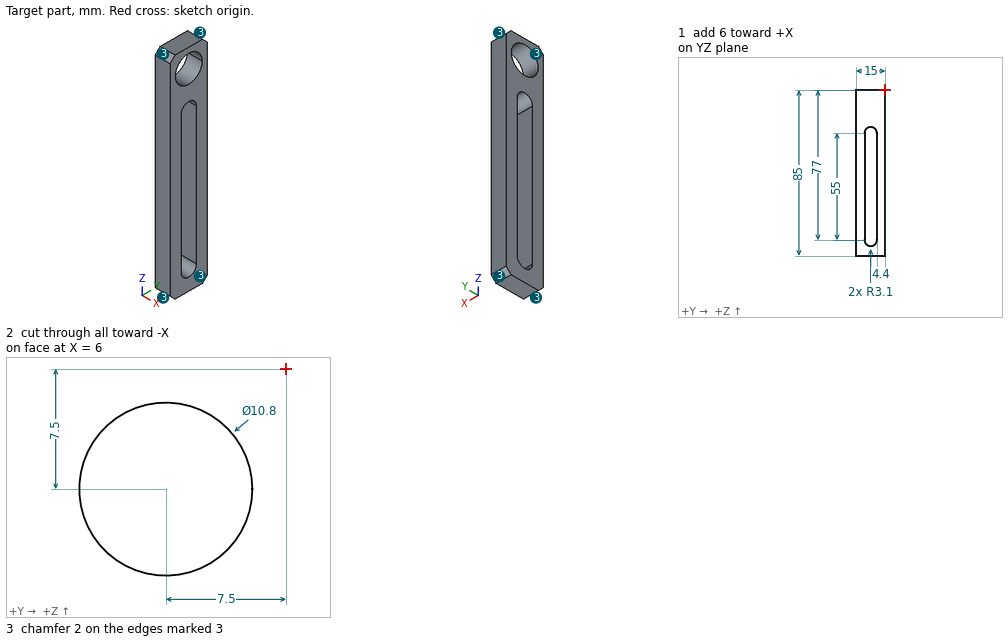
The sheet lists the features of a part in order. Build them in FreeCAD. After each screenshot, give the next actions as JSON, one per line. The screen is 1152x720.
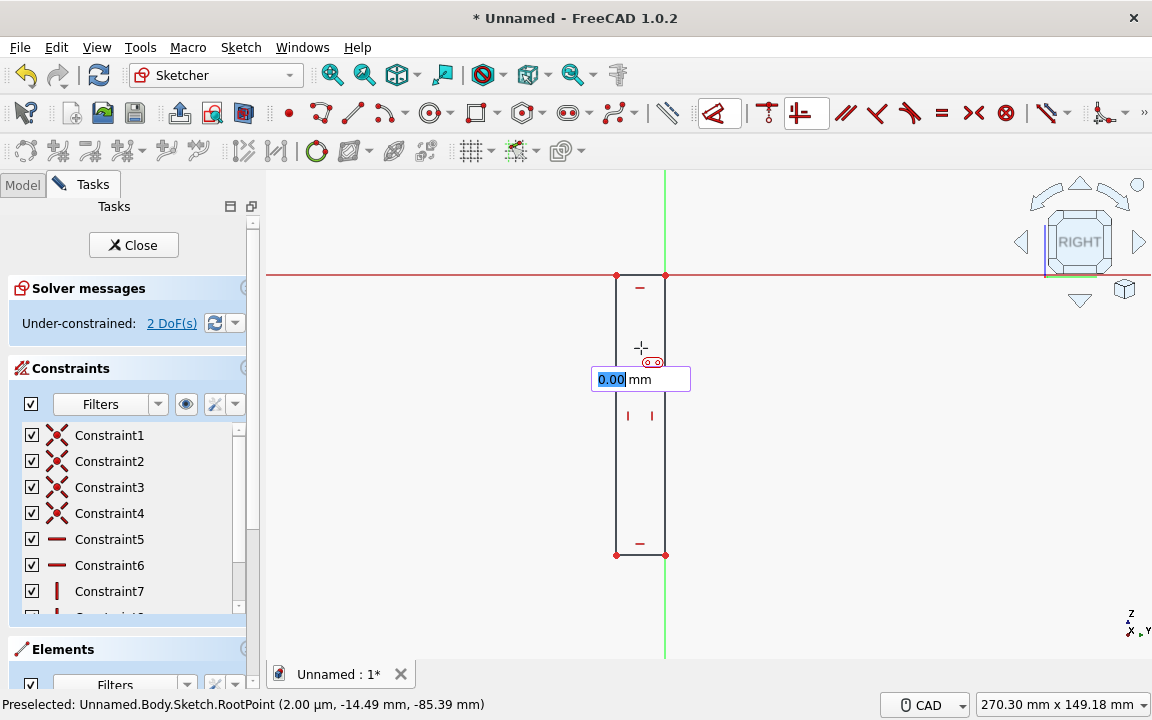
{"action": "scroll", "coordinate": [651, 438], "scroll_direction": "up", "scroll_amount": 3}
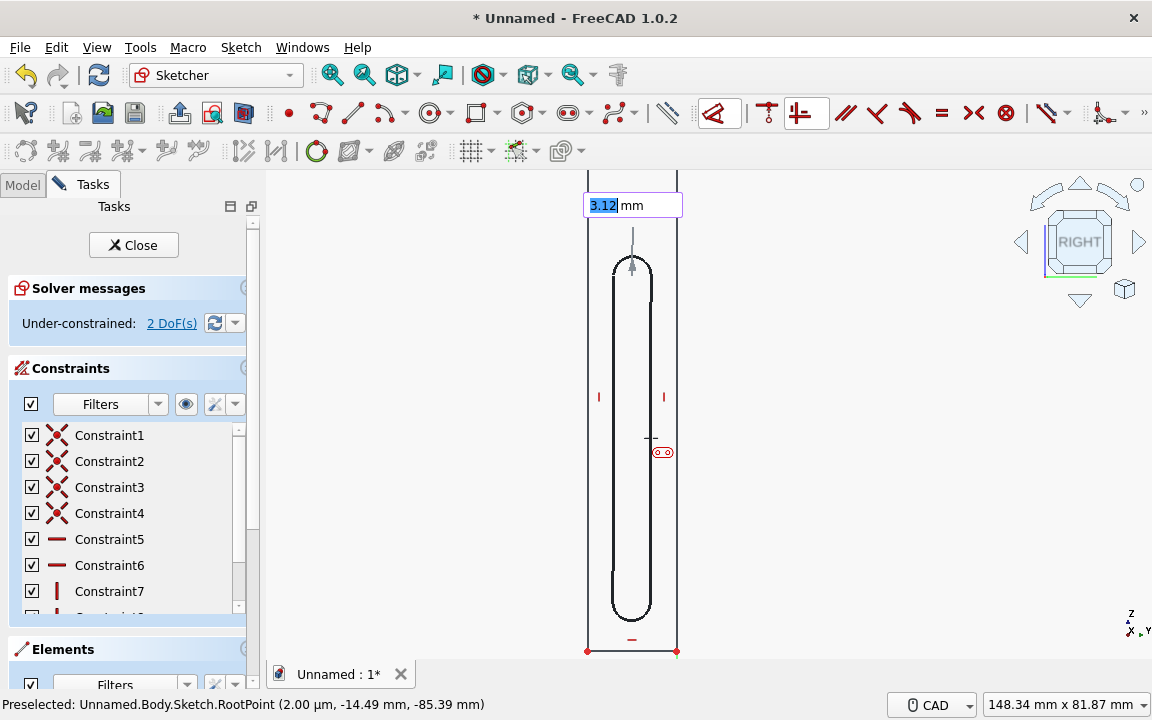
{"action": "left_click", "coordinate": [650, 437]}
{"action": "key", "text": "Escape"}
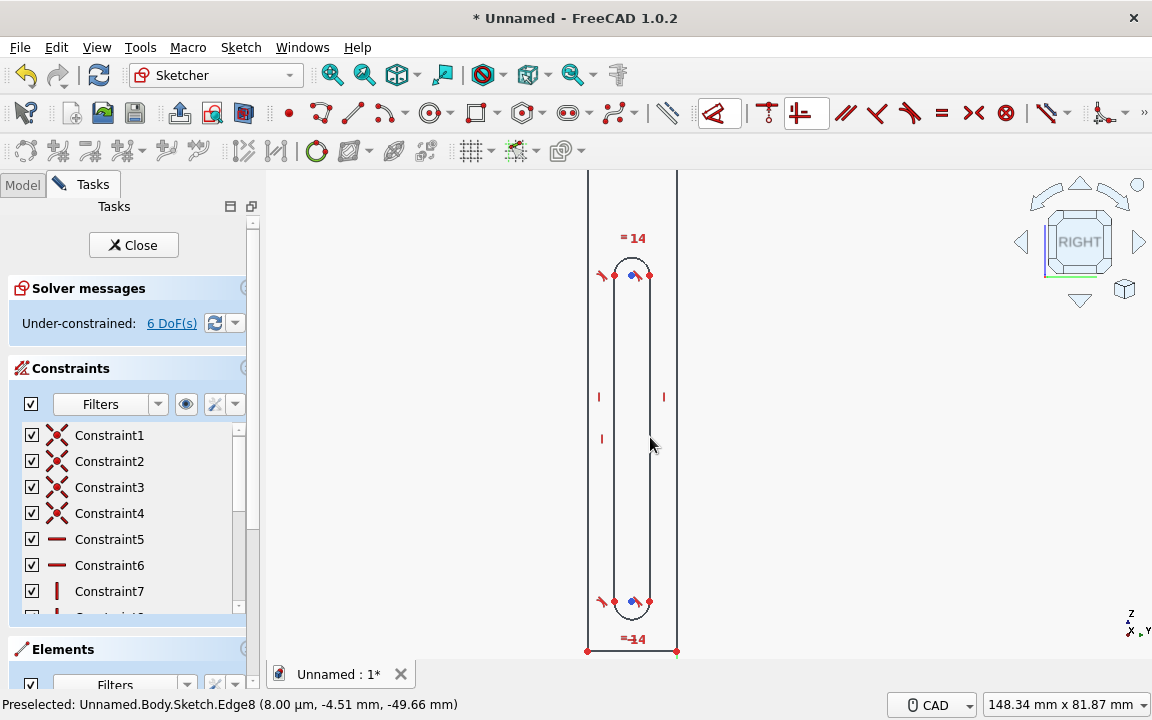
{"action": "left_click", "coordinate": [714, 114]}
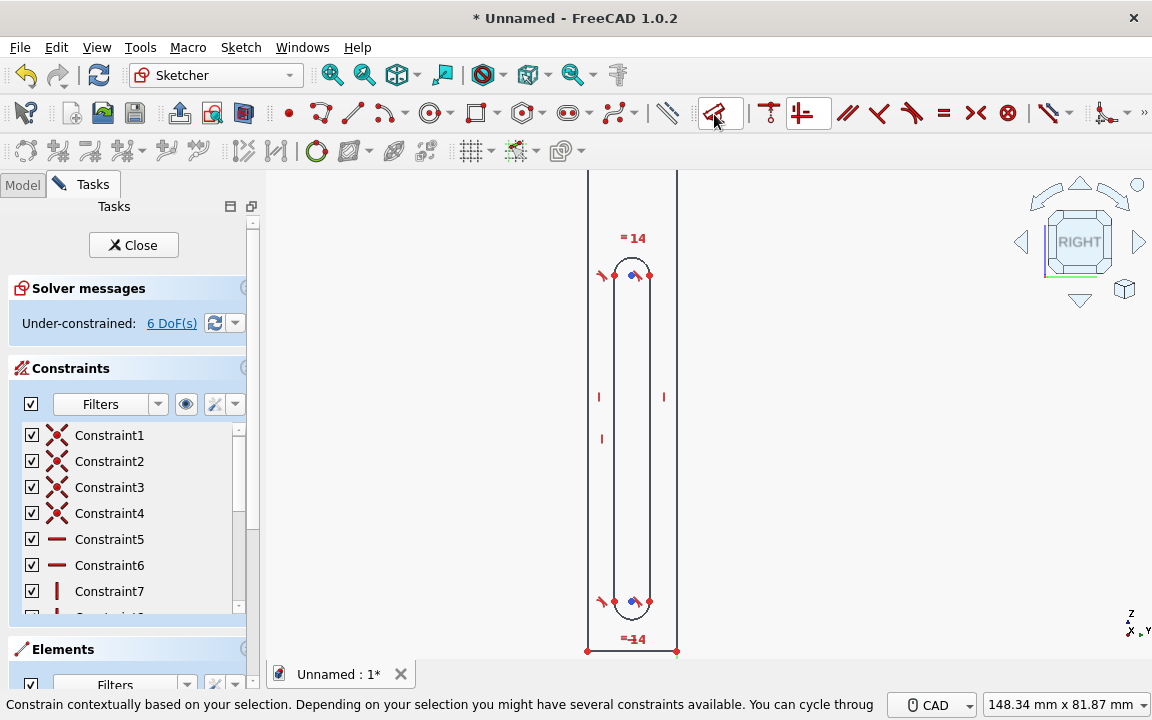
{"action": "scroll", "coordinate": [622, 616], "scroll_direction": "up", "scroll_amount": 4}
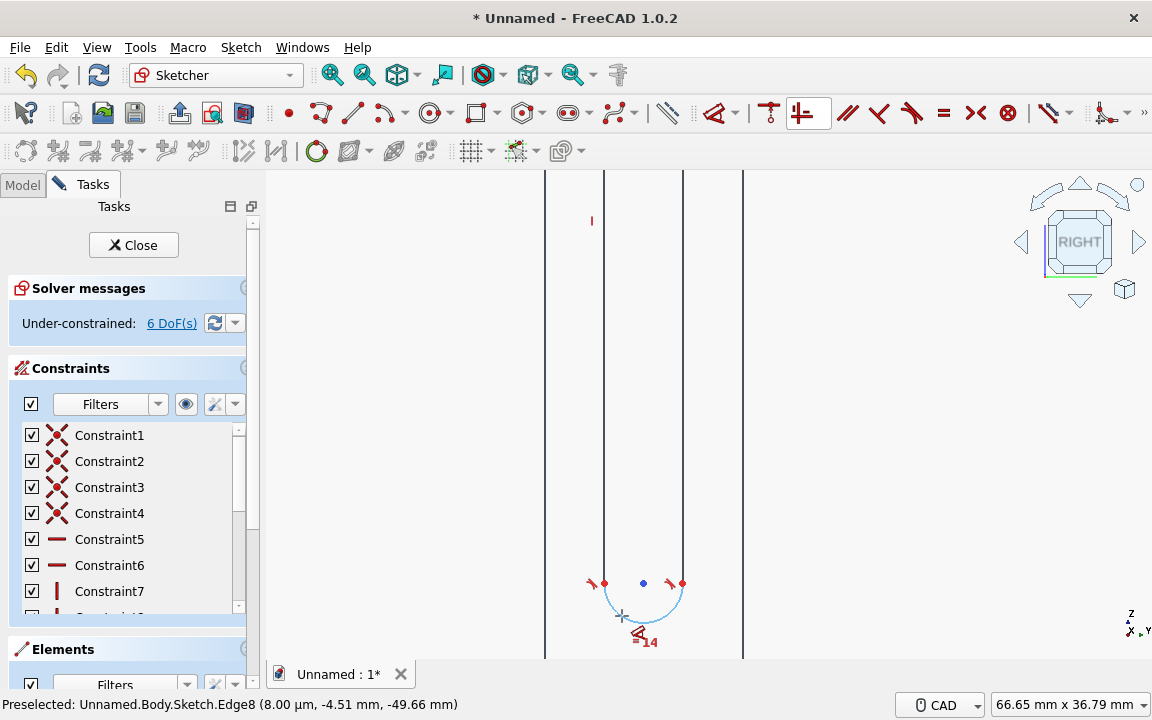
{"action": "left_click", "coordinate": [621, 615]}
{"action": "left_click", "coordinate": [580, 614]}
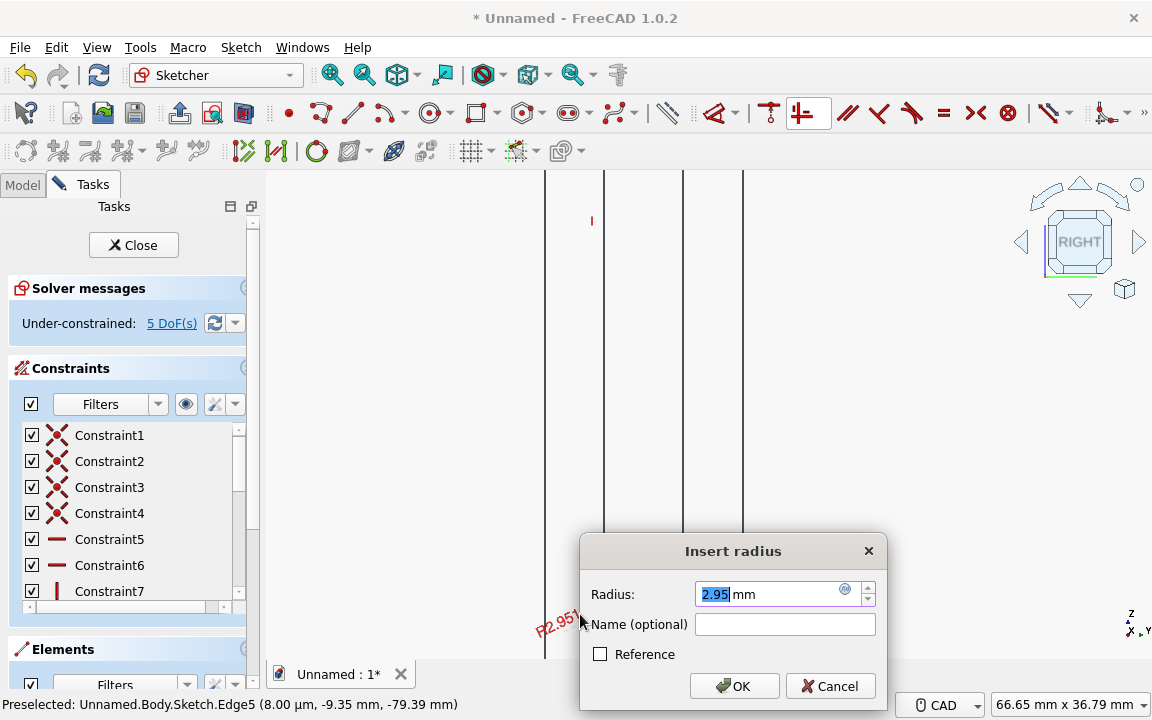
{"action": "type", "text": "3.1"}
{"action": "key", "text": "Return"}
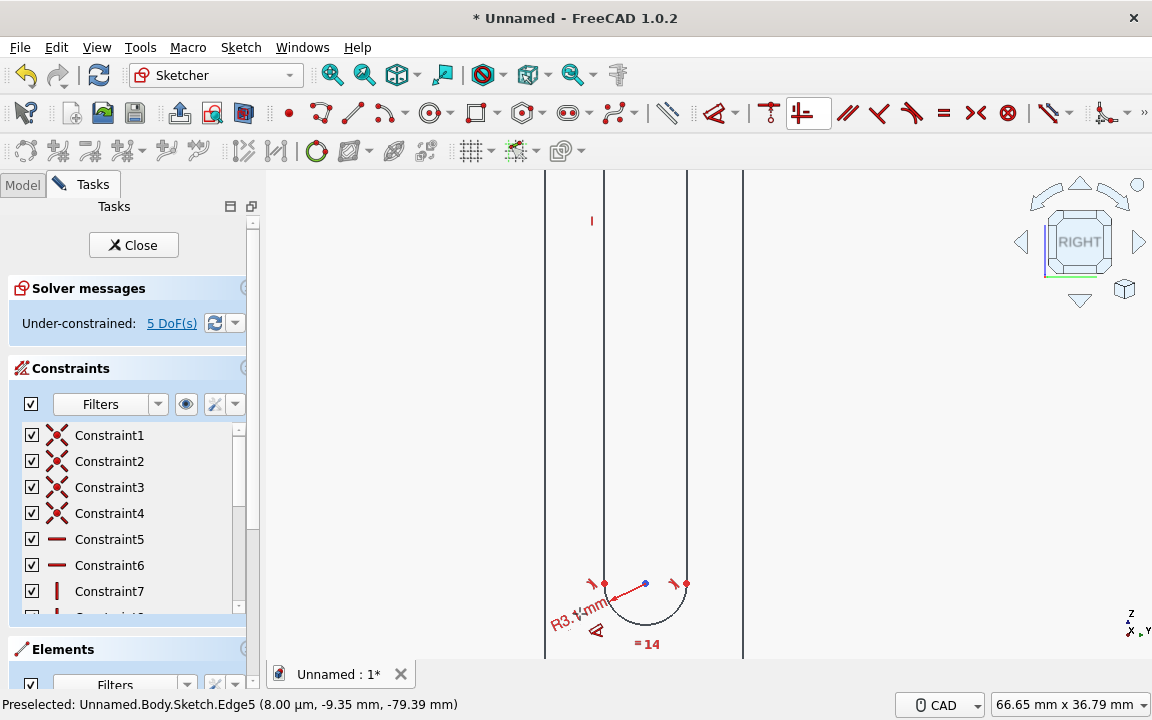
{"action": "scroll", "coordinate": [640, 510], "scroll_direction": "down", "scroll_amount": 7}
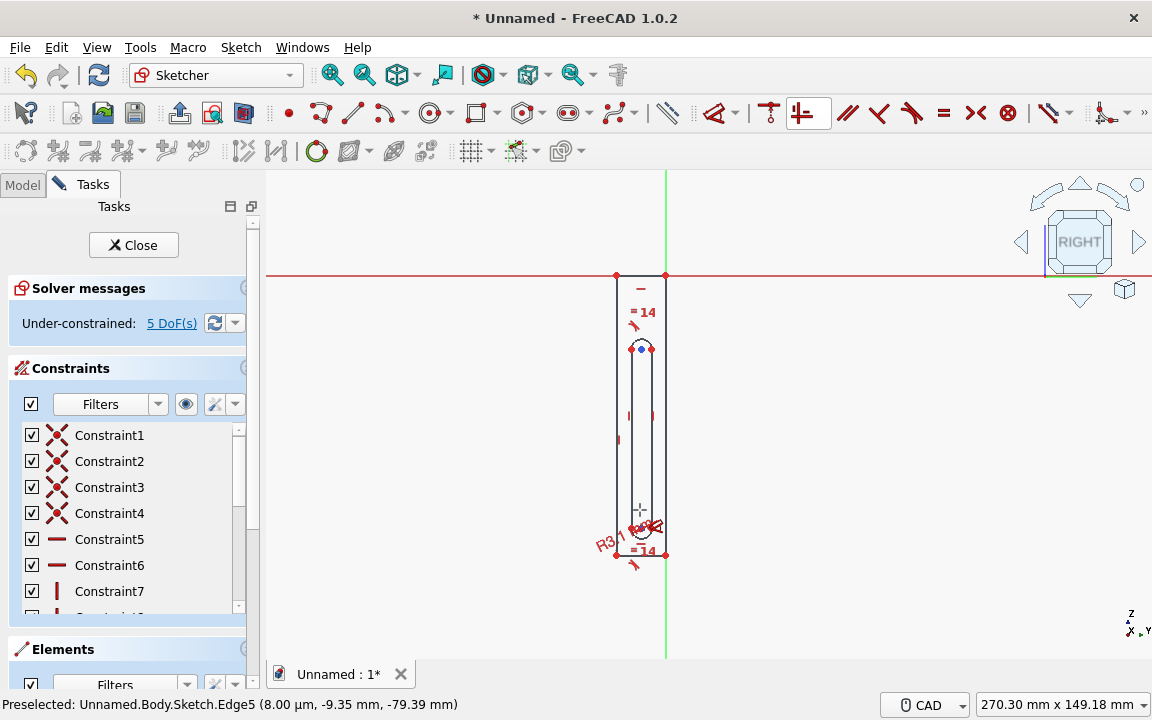
{"action": "left_click", "coordinate": [651, 276]}
{"action": "left_click", "coordinate": [641, 242]}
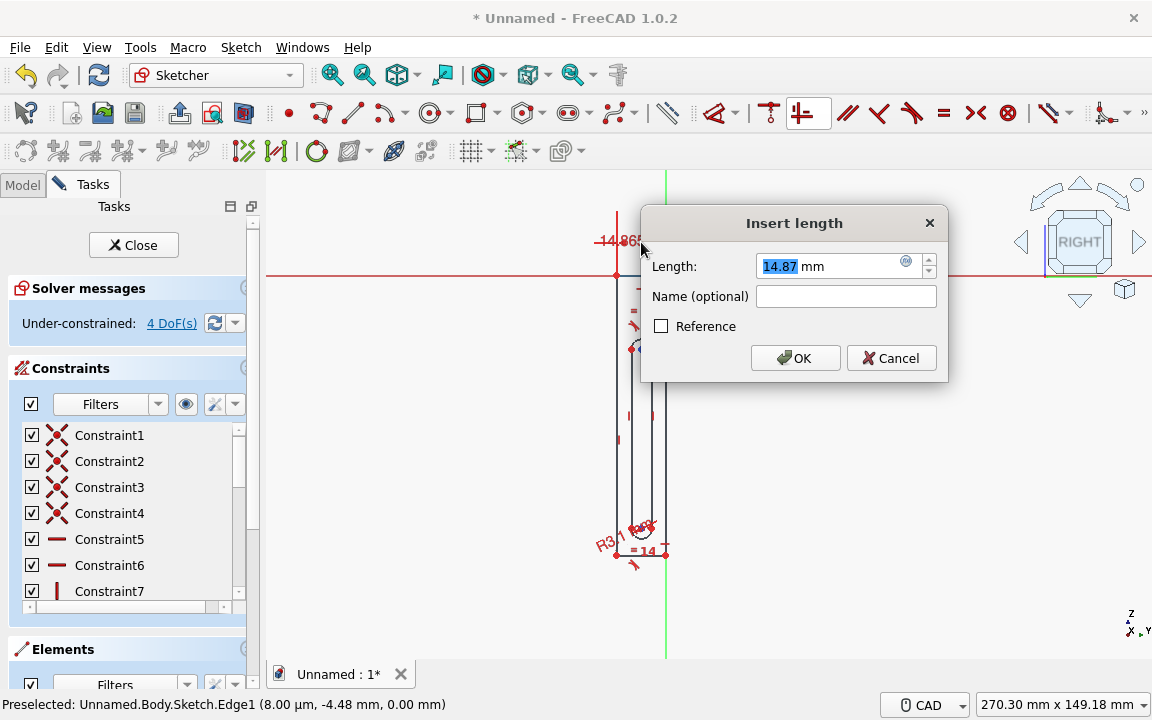
{"action": "type", "text": "15"}
{"action": "key", "text": "Return"}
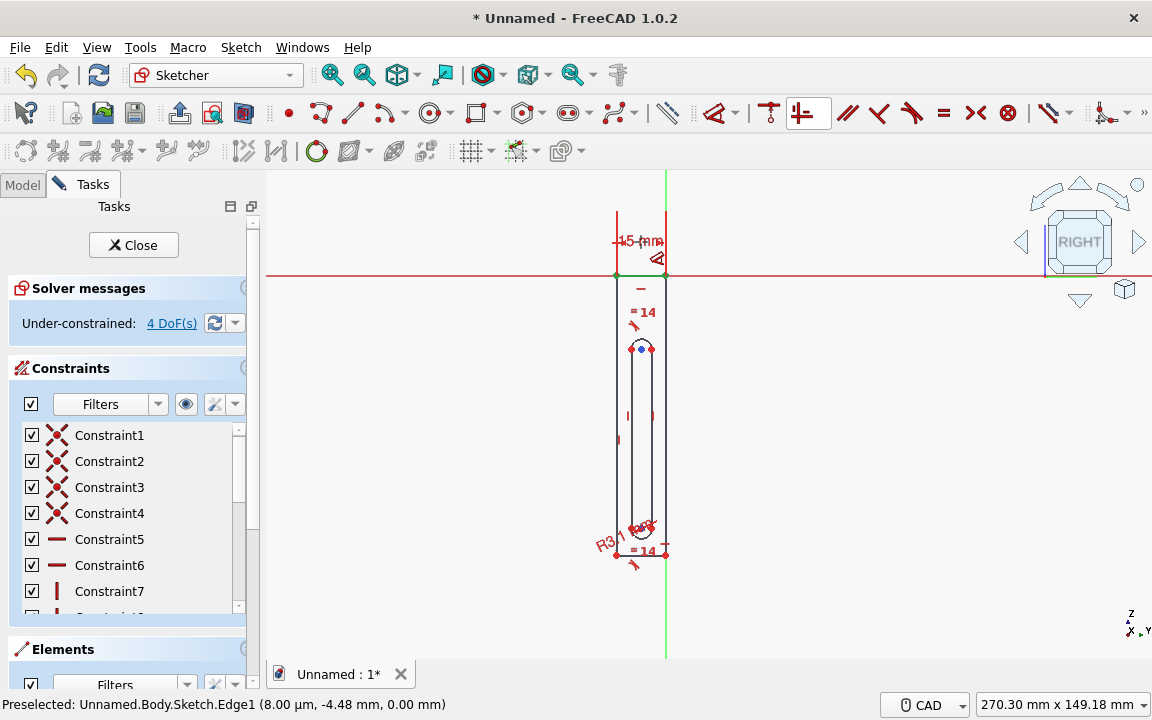
{"action": "left_click", "coordinate": [617, 360]}
{"action": "left_click", "coordinate": [583, 416]}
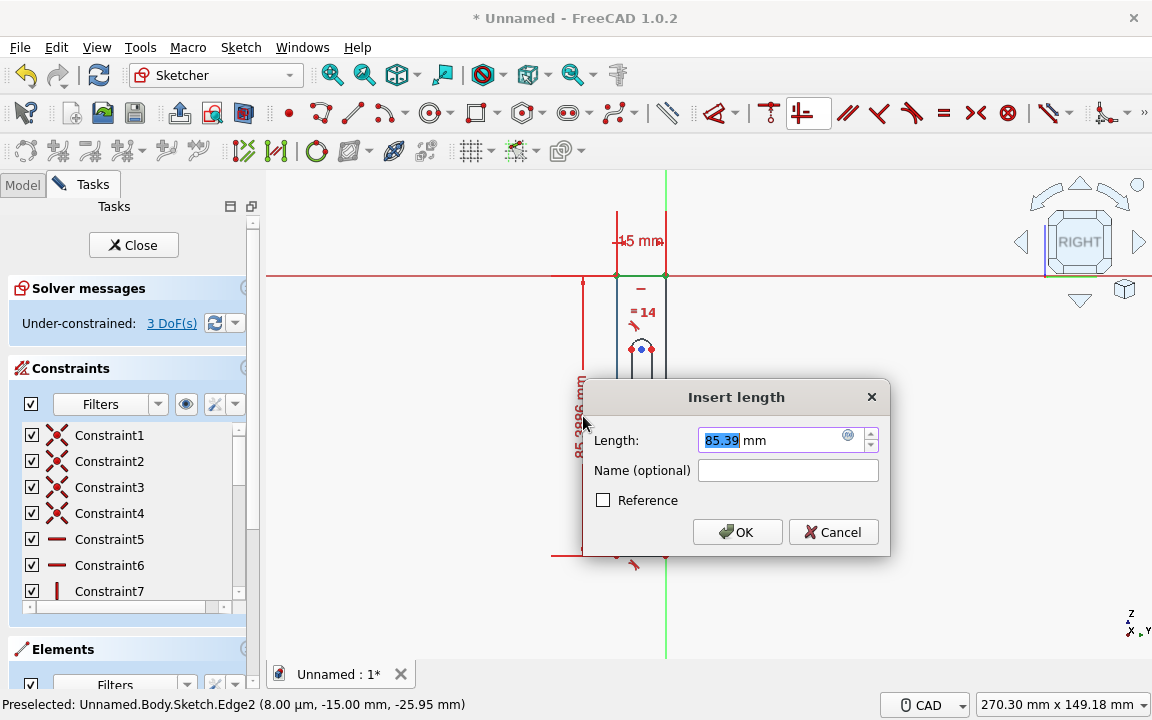
{"action": "type", "text": "85"}
{"action": "key", "text": "Return"}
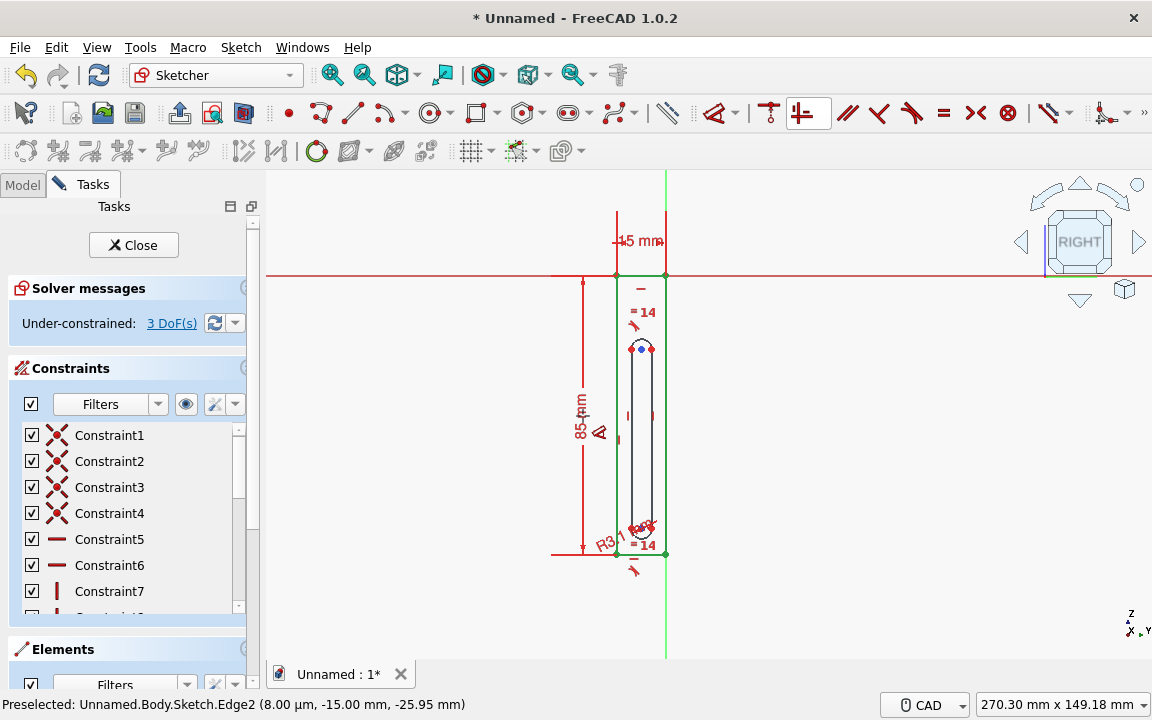
{"action": "left_click", "coordinate": [632, 475]}
{"action": "left_click", "coordinate": [598, 439]}